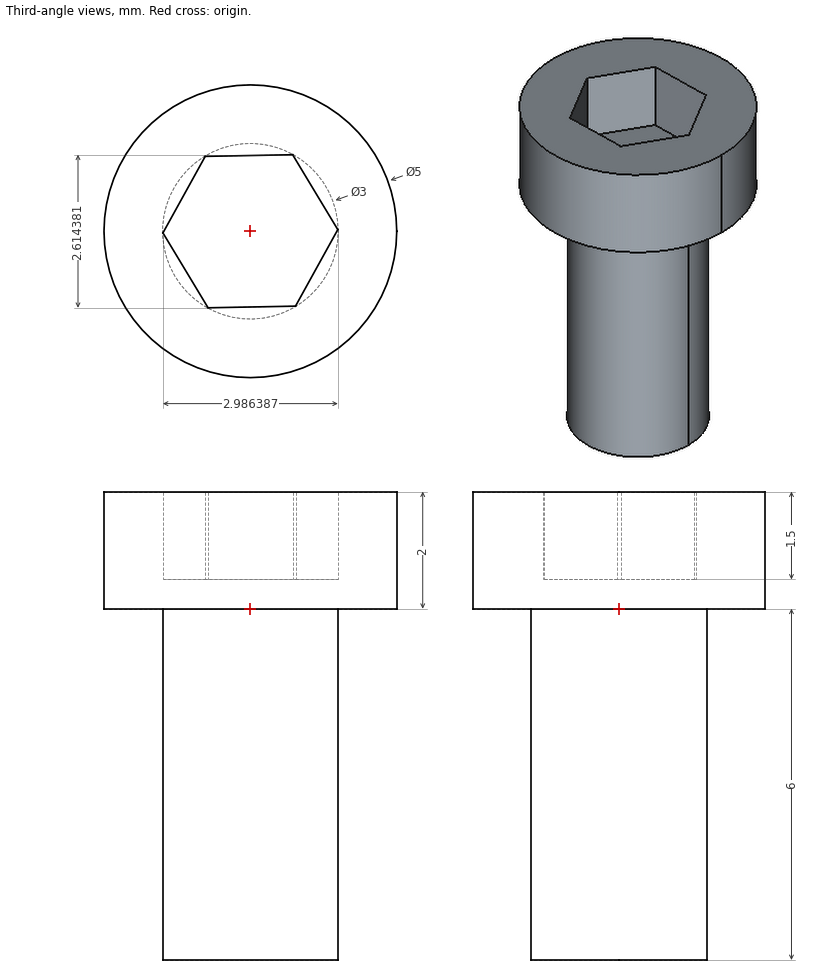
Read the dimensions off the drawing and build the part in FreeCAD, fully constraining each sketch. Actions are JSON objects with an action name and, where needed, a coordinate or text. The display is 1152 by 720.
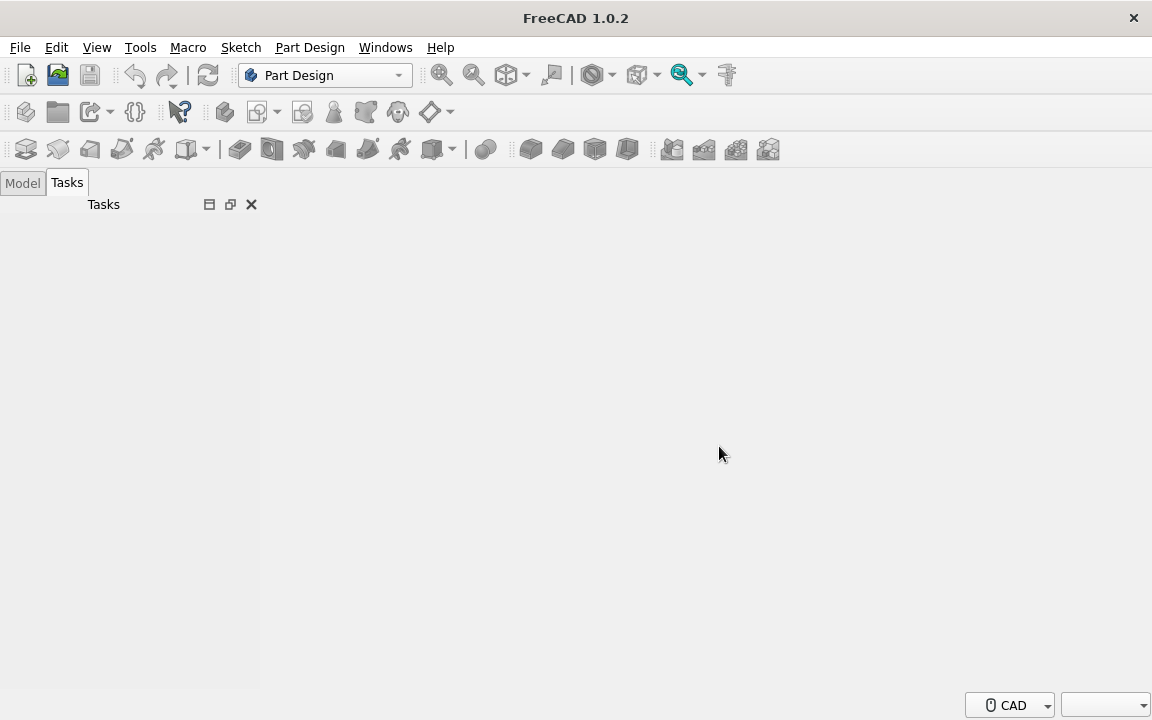
{"action": "left_click", "coordinate": [26, 76]}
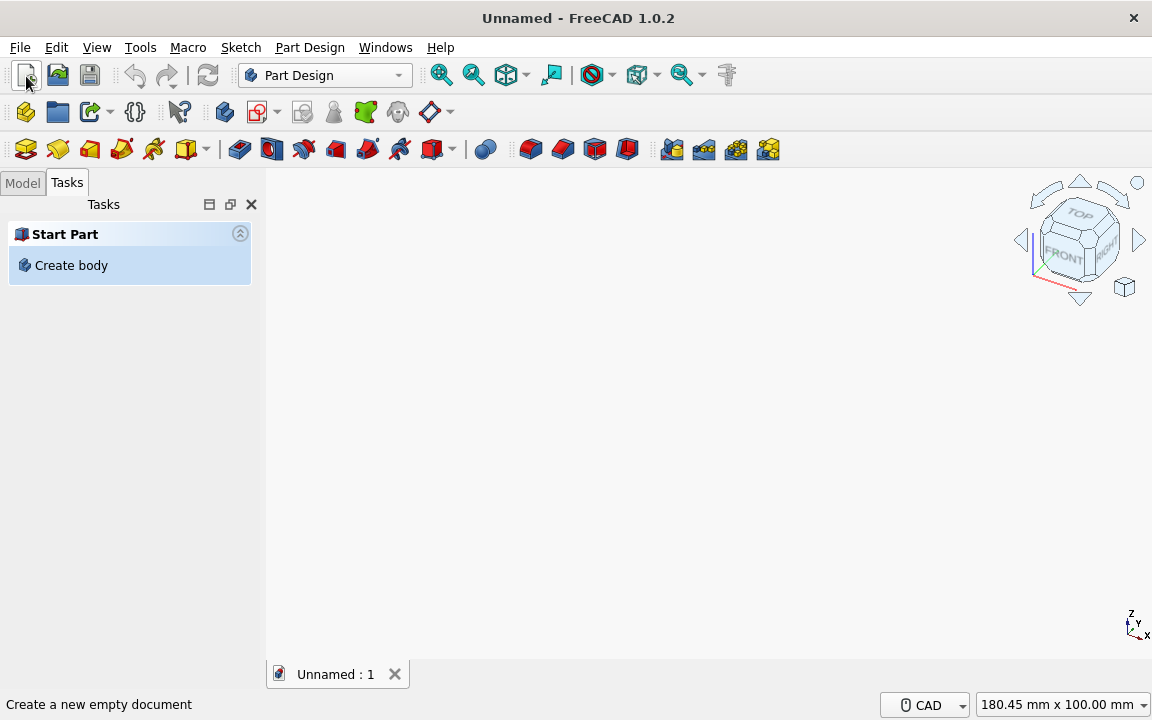
{"action": "left_click", "coordinate": [258, 112]}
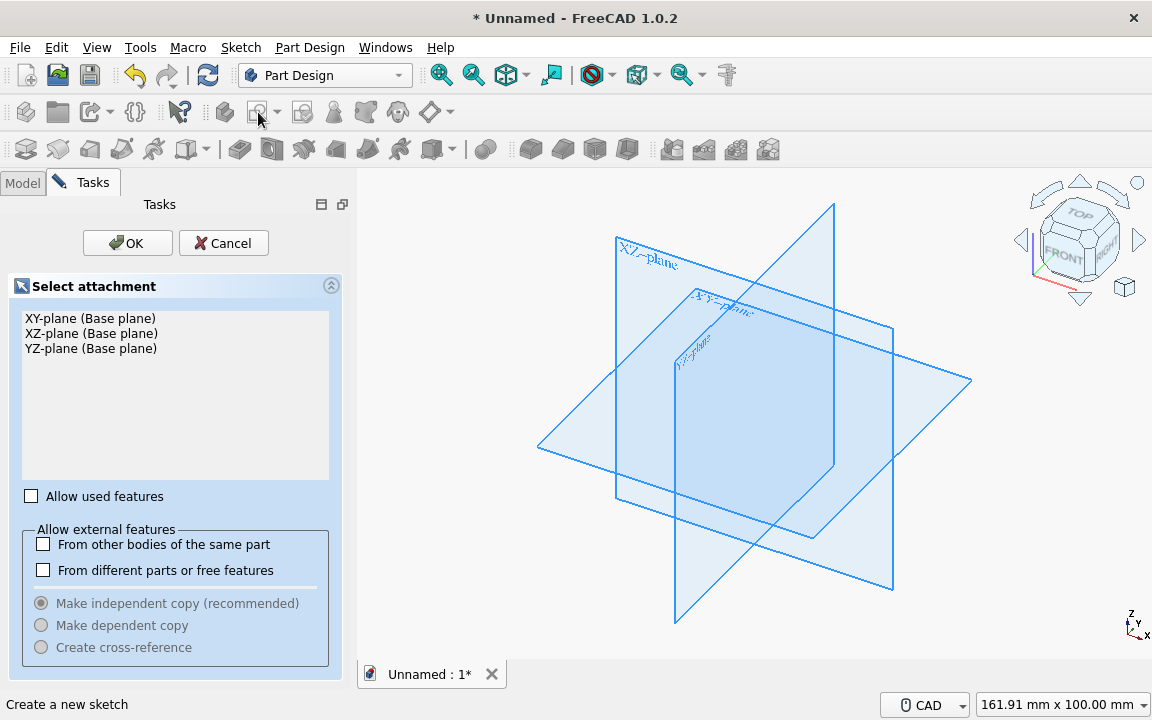
{"action": "left_click", "coordinate": [82, 318]}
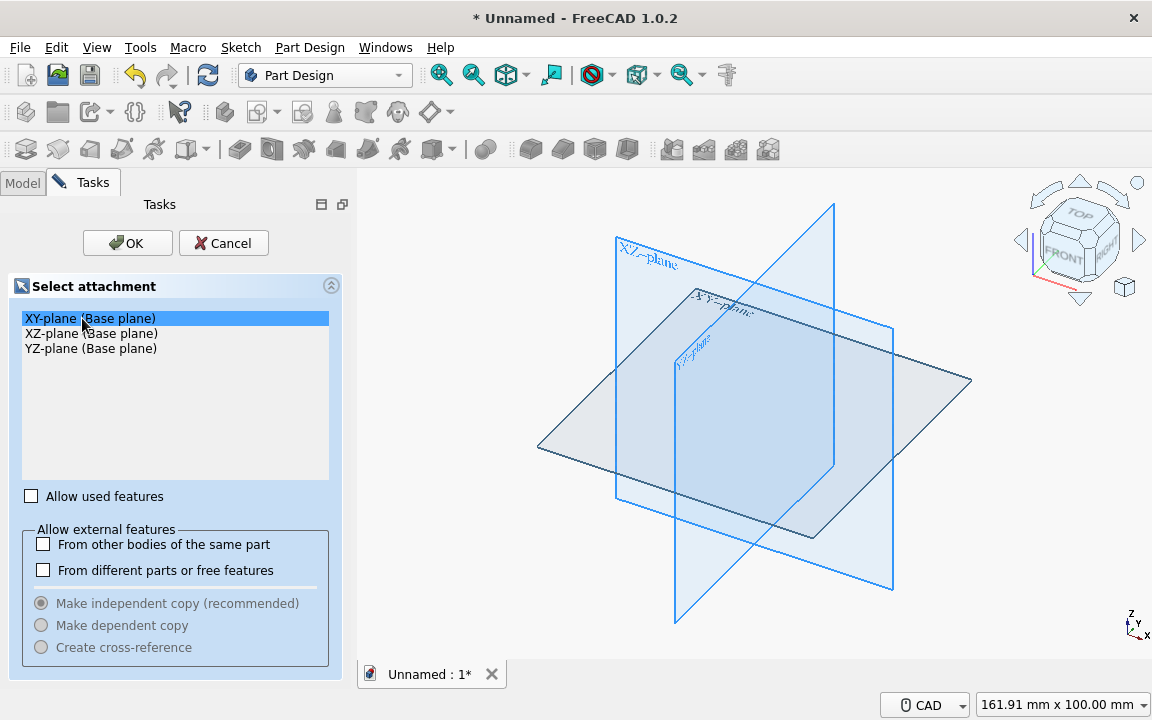
{"action": "left_click", "coordinate": [128, 243]}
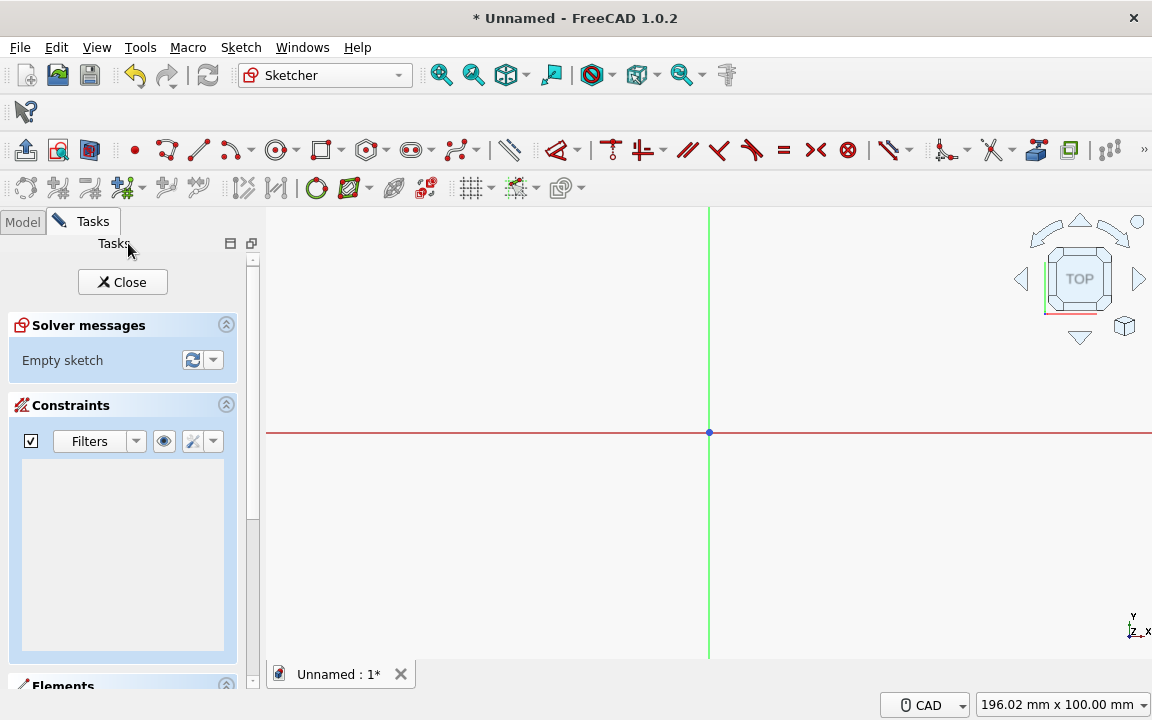
{"action": "scroll", "coordinate": [713, 433], "scroll_direction": "up", "scroll_amount": 15}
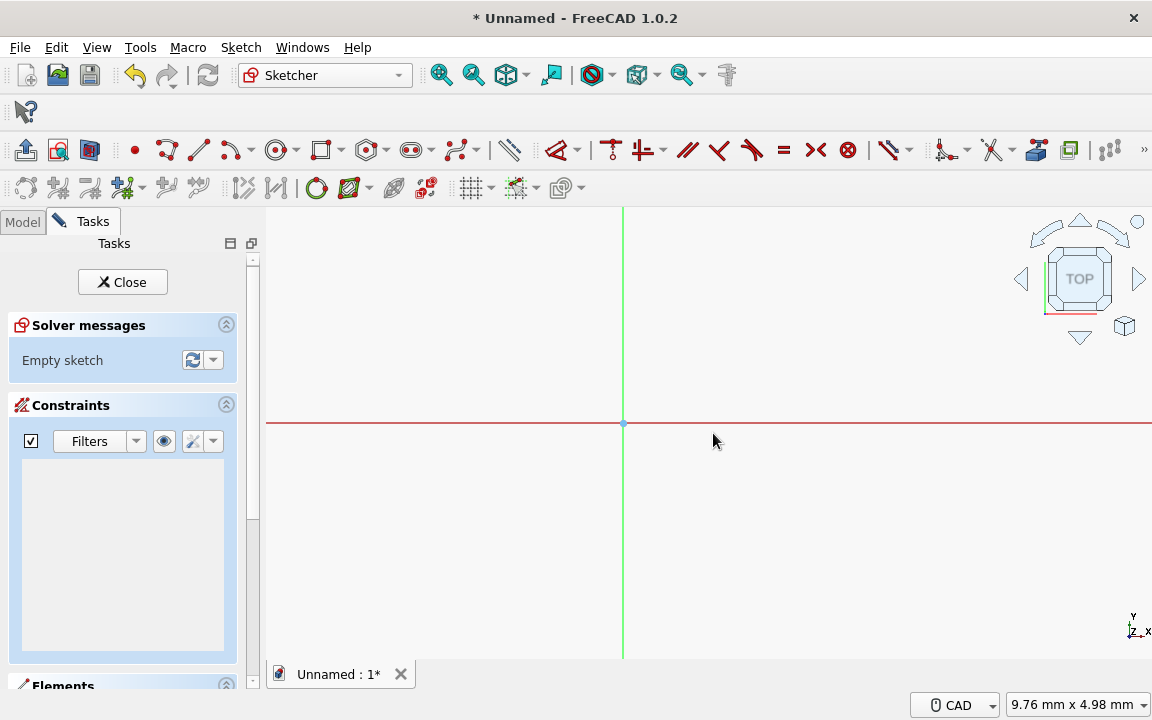
{"action": "key", "text": "g c"}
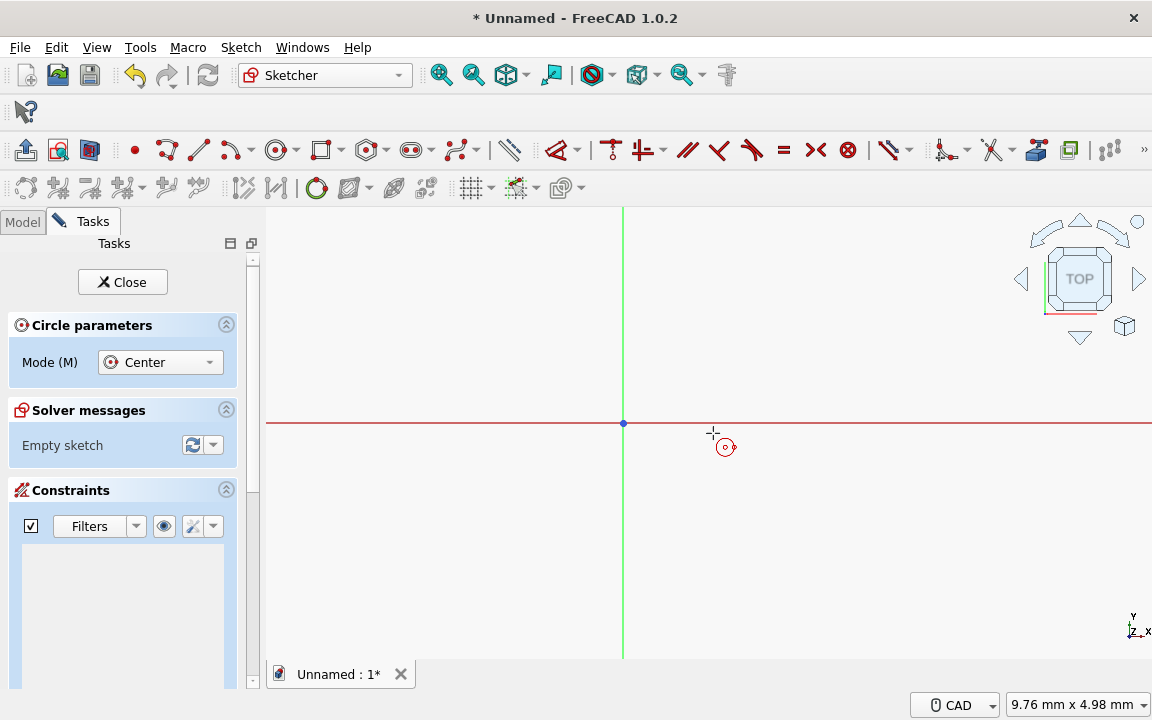
{"action": "left_click", "coordinate": [623, 423]}
{"action": "mouse_move", "coordinate": [719, 327]}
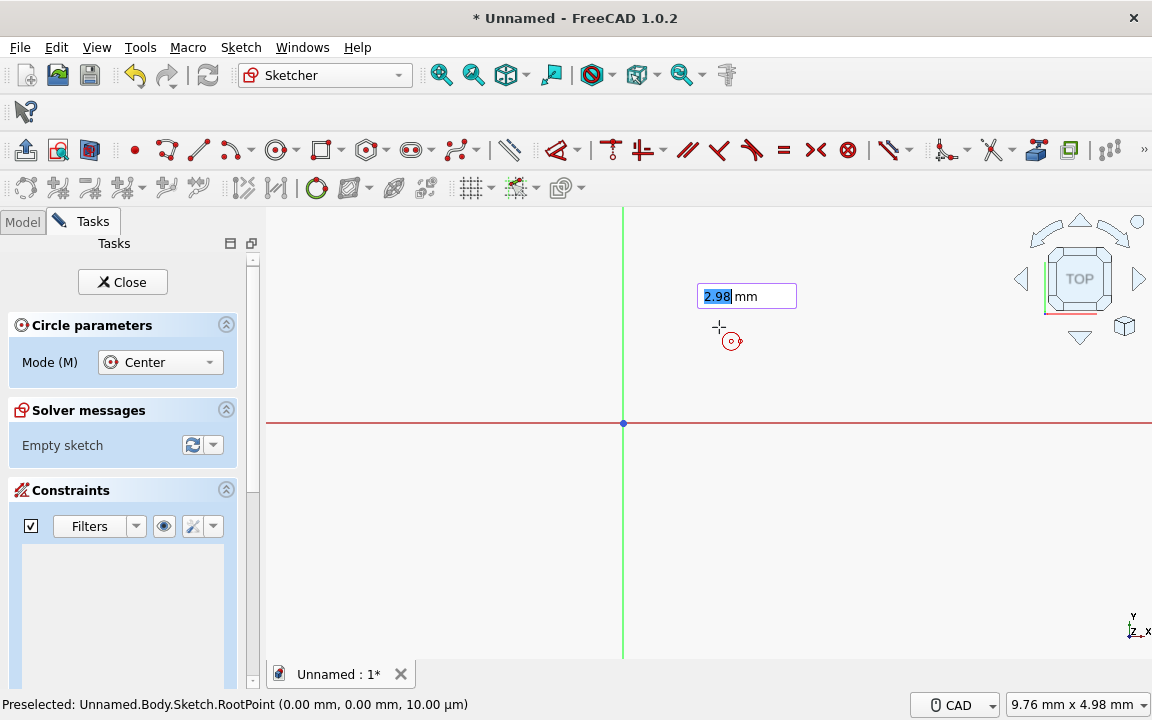
{"action": "type", "text": "3"}
{"action": "key", "text": "Return"}
{"action": "key", "text": "Escape"}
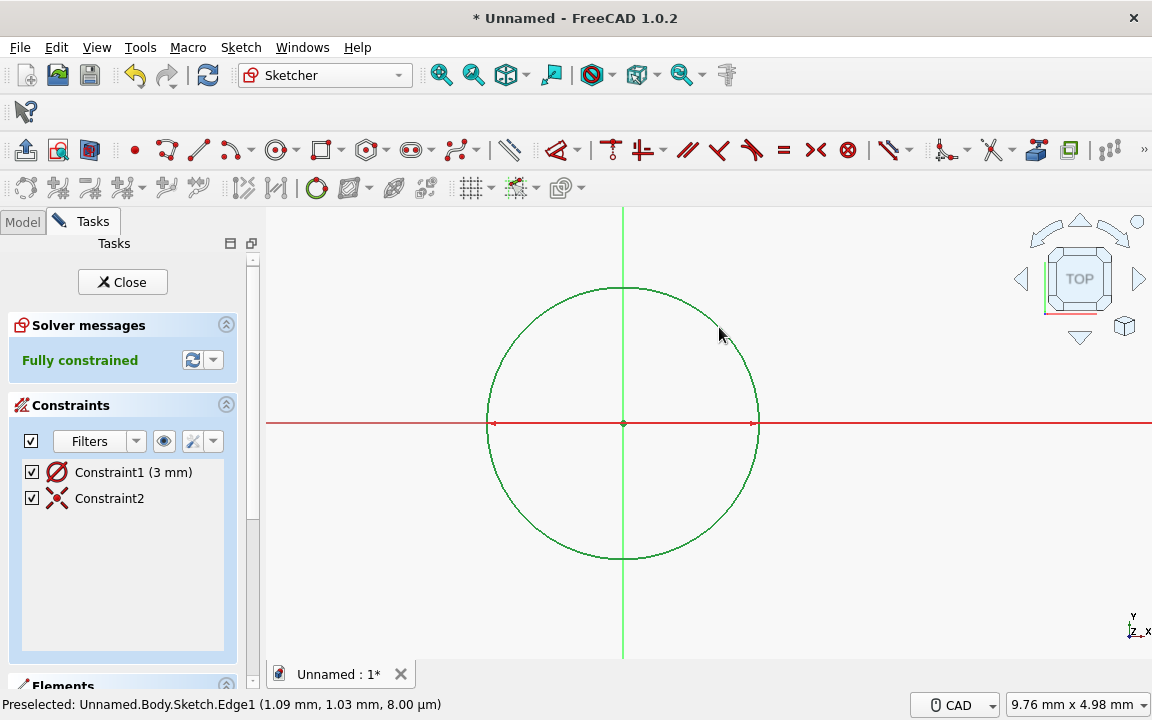
{"action": "left_click", "coordinate": [123, 282]}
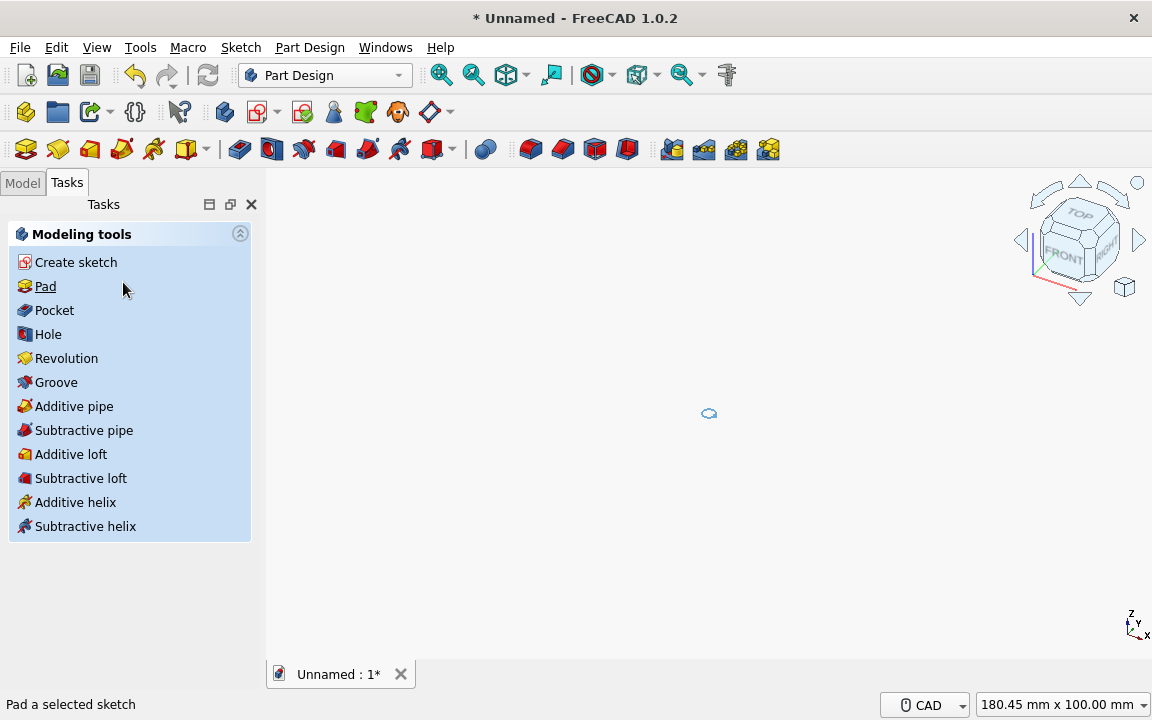
{"action": "left_click", "coordinate": [26, 150]}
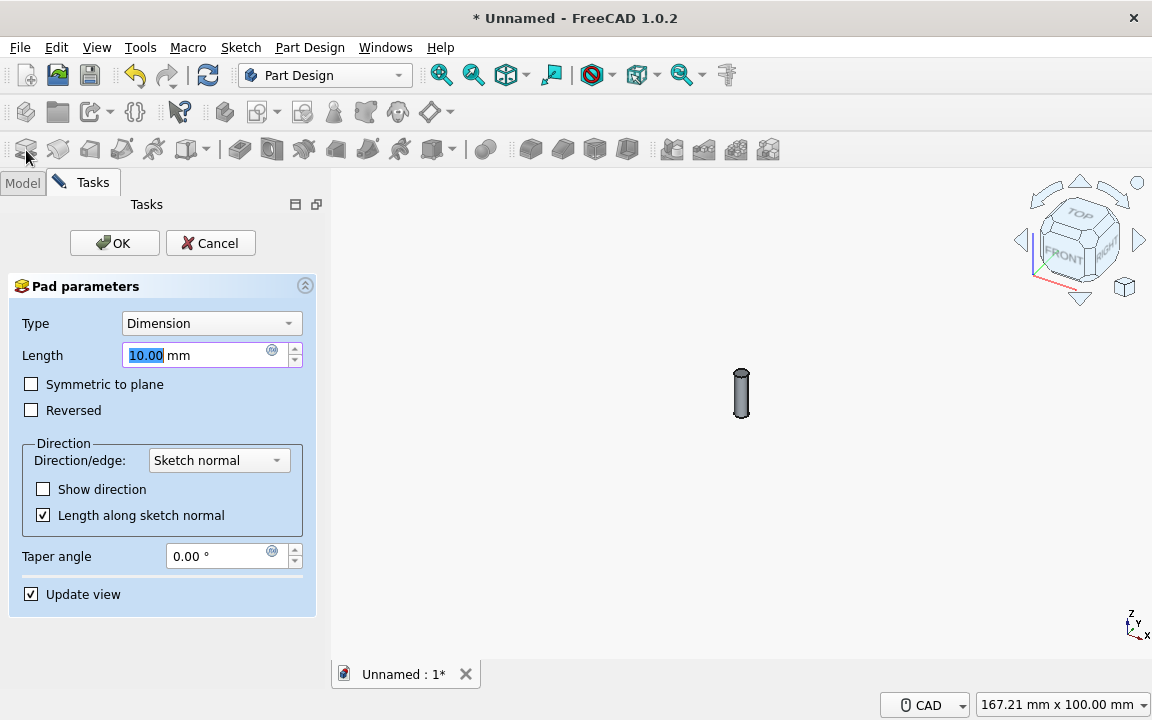
{"action": "type", "text": "6"}
{"action": "key", "text": "Tab"}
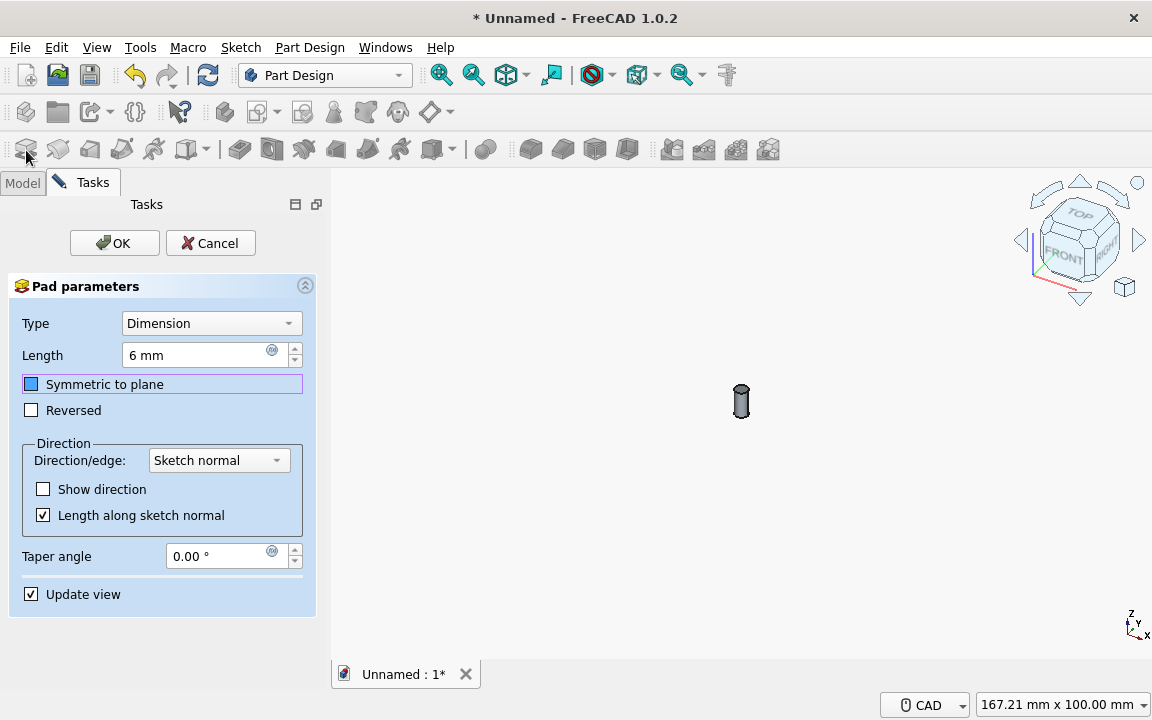
{"action": "left_click", "coordinate": [30, 410]}